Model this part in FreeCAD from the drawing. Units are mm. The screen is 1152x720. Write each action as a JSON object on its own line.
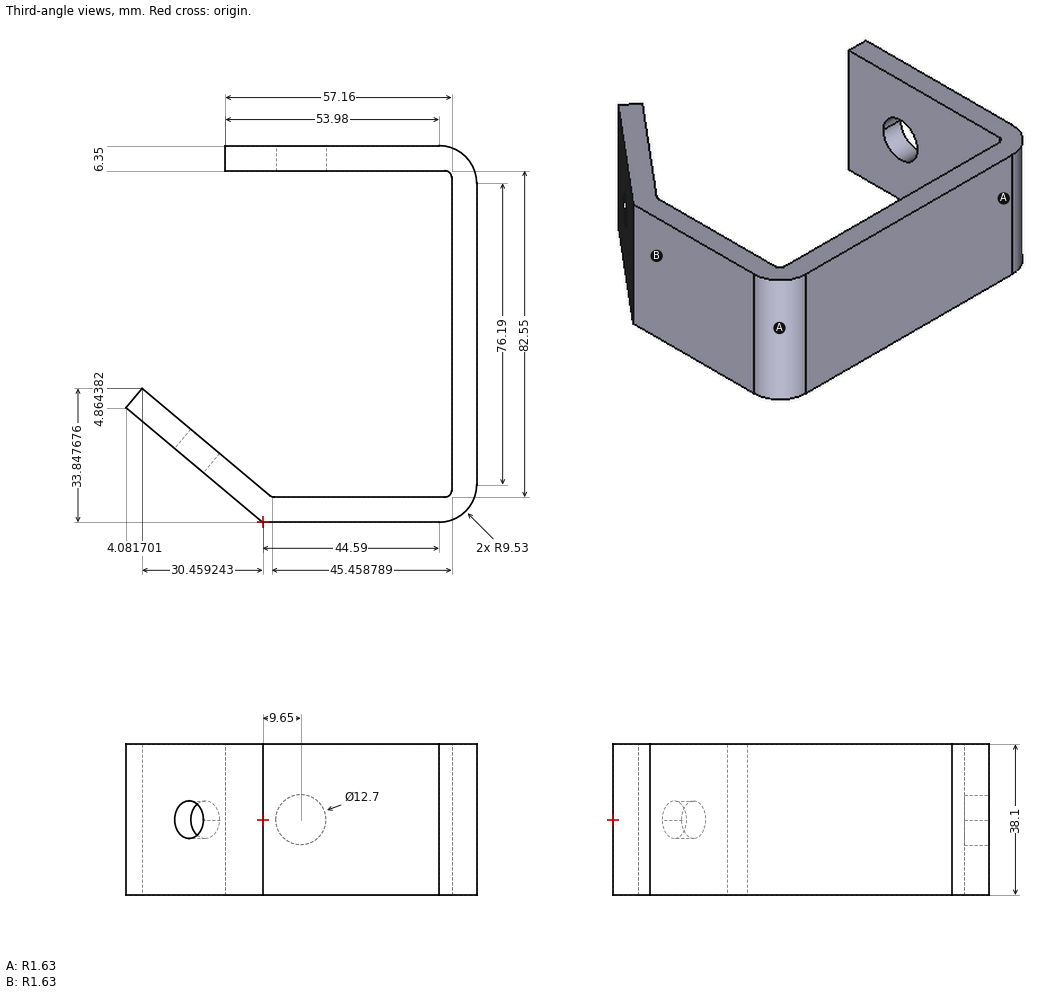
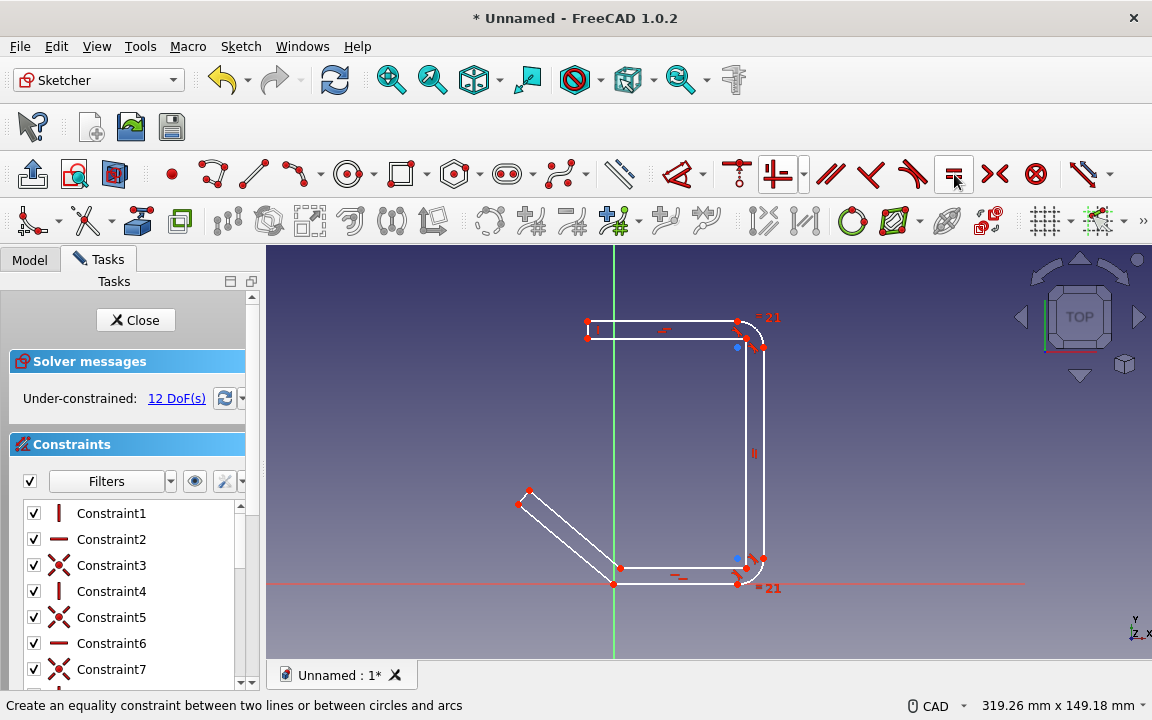
{"action": "key", "text": "d"}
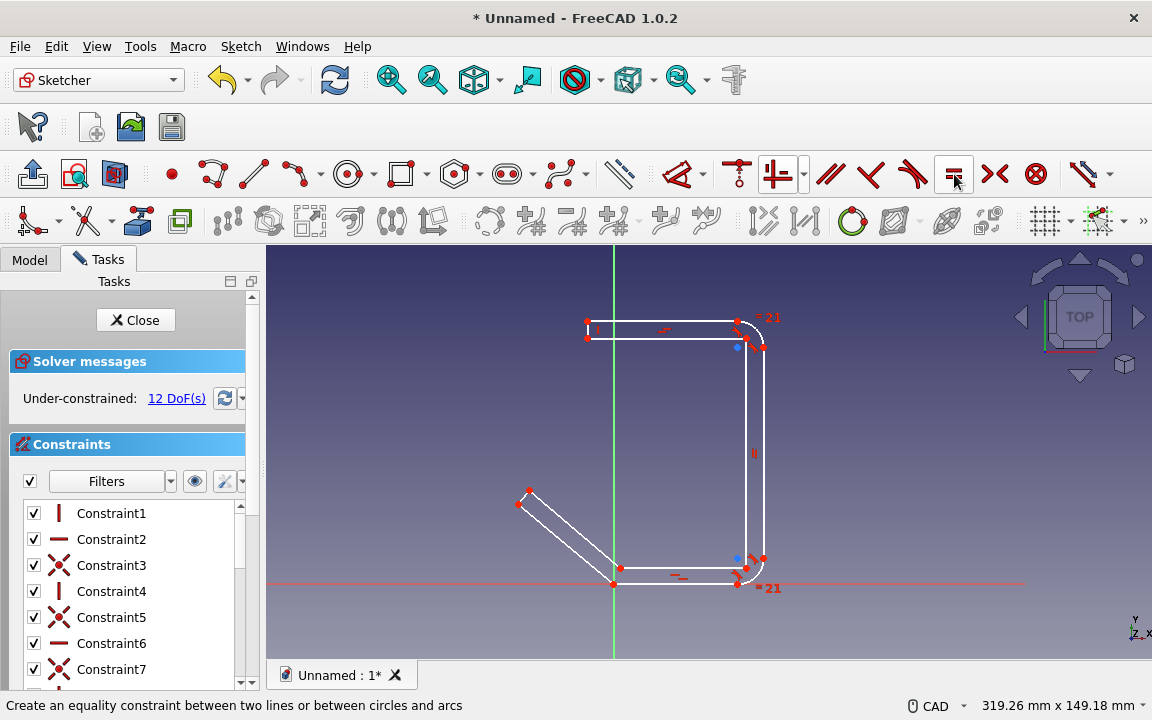
{"action": "scroll", "coordinate": [761, 335], "scroll_direction": "up", "scroll_amount": 3}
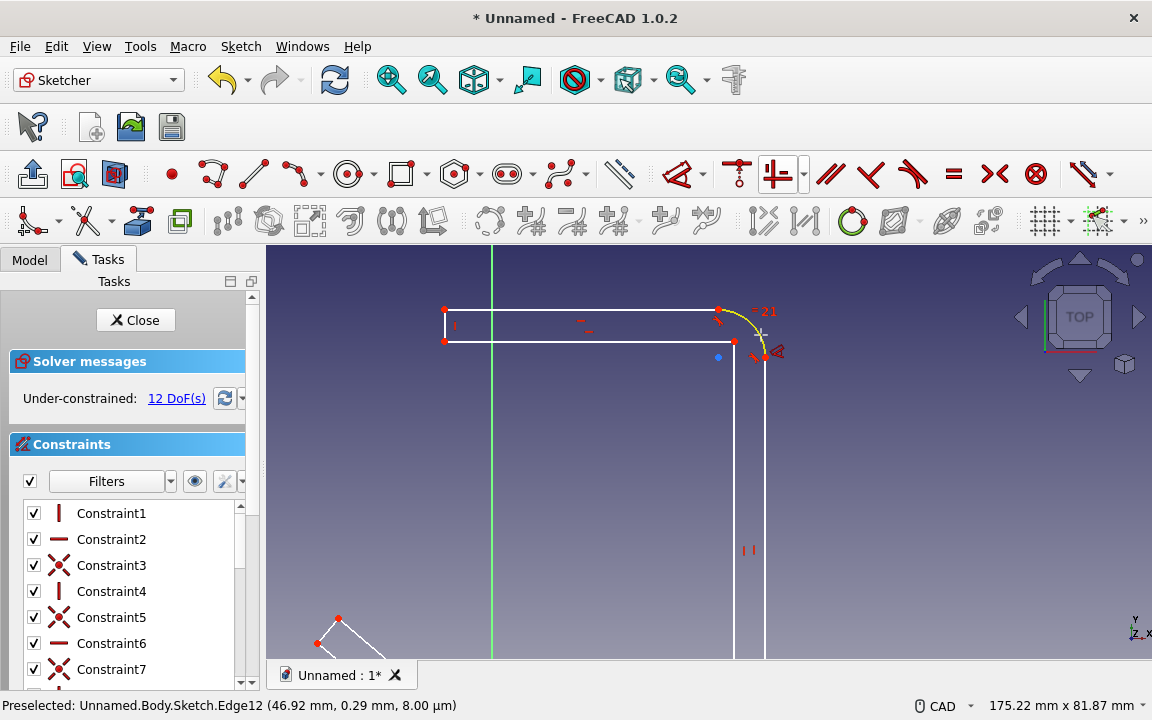
{"action": "left_click", "coordinate": [760, 336]}
{"action": "left_click", "coordinate": [789, 322]}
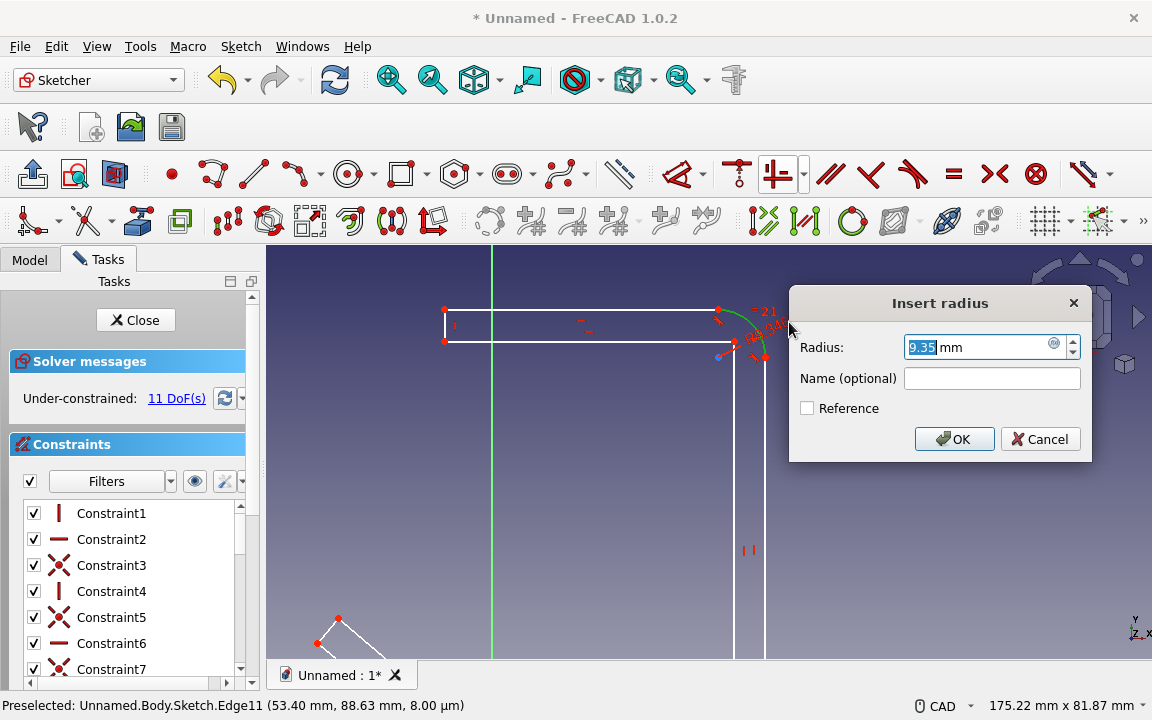
{"action": "type", "text": "9.53"}
{"action": "key", "text": "Return"}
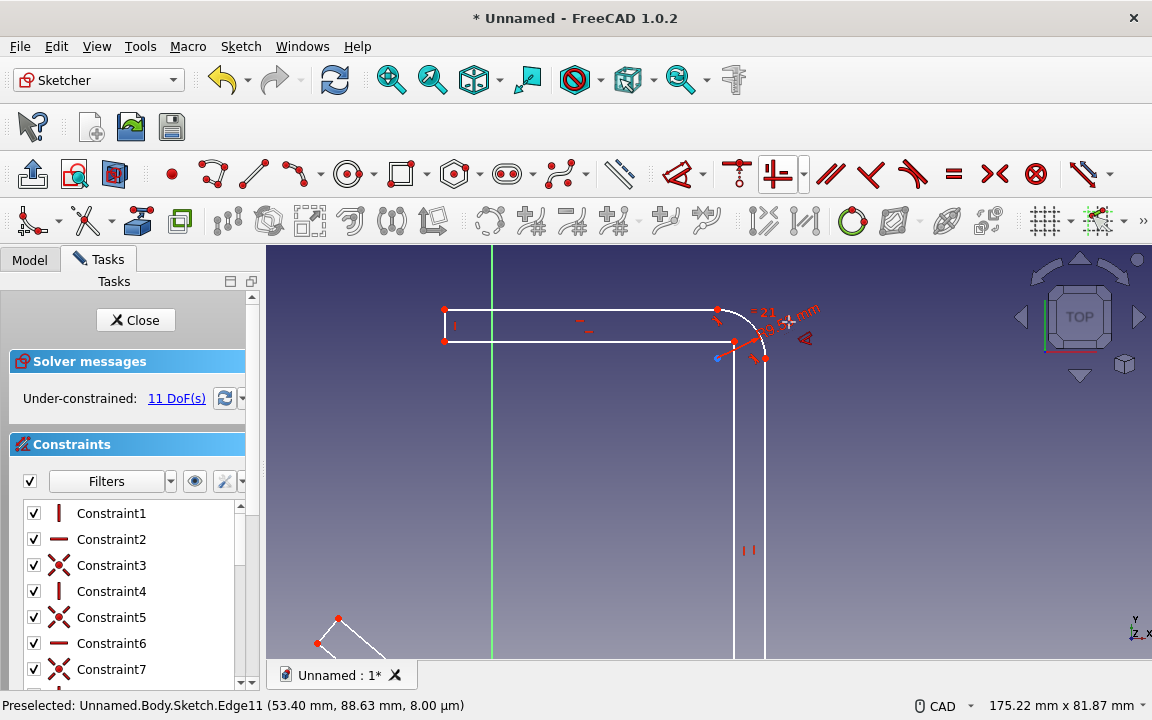
{"action": "scroll", "coordinate": [445, 319], "scroll_direction": "up", "scroll_amount": 2}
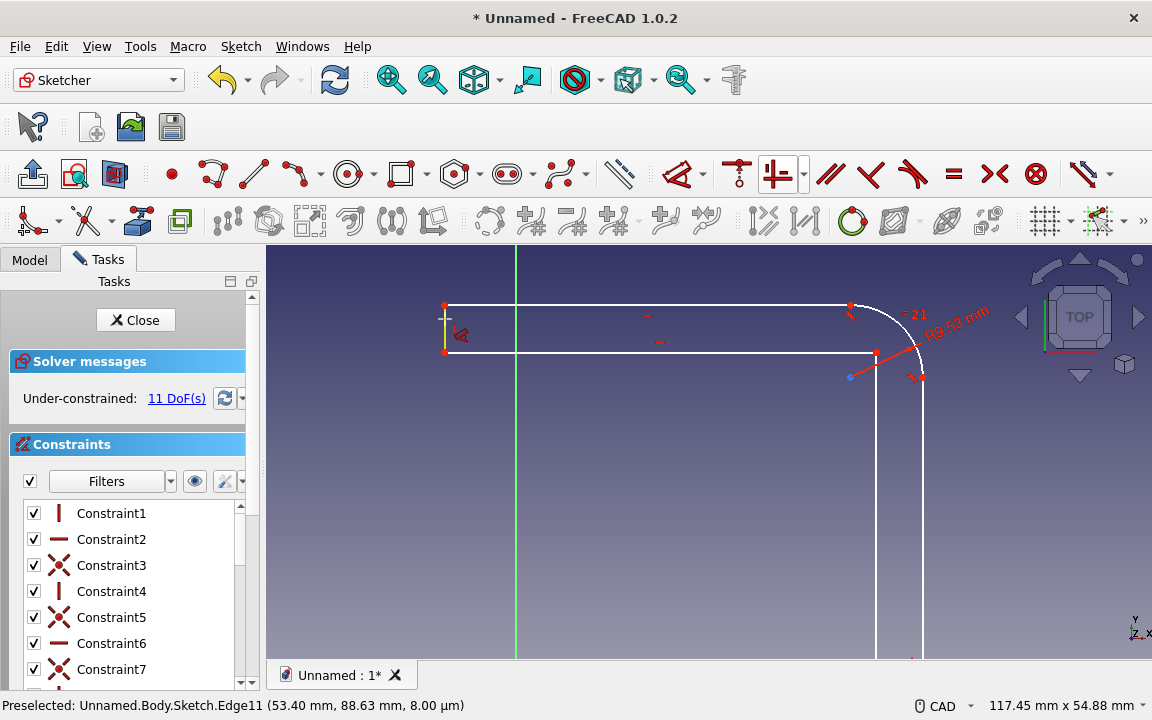
{"action": "left_click", "coordinate": [445, 319]}
{"action": "left_click", "coordinate": [411, 329]}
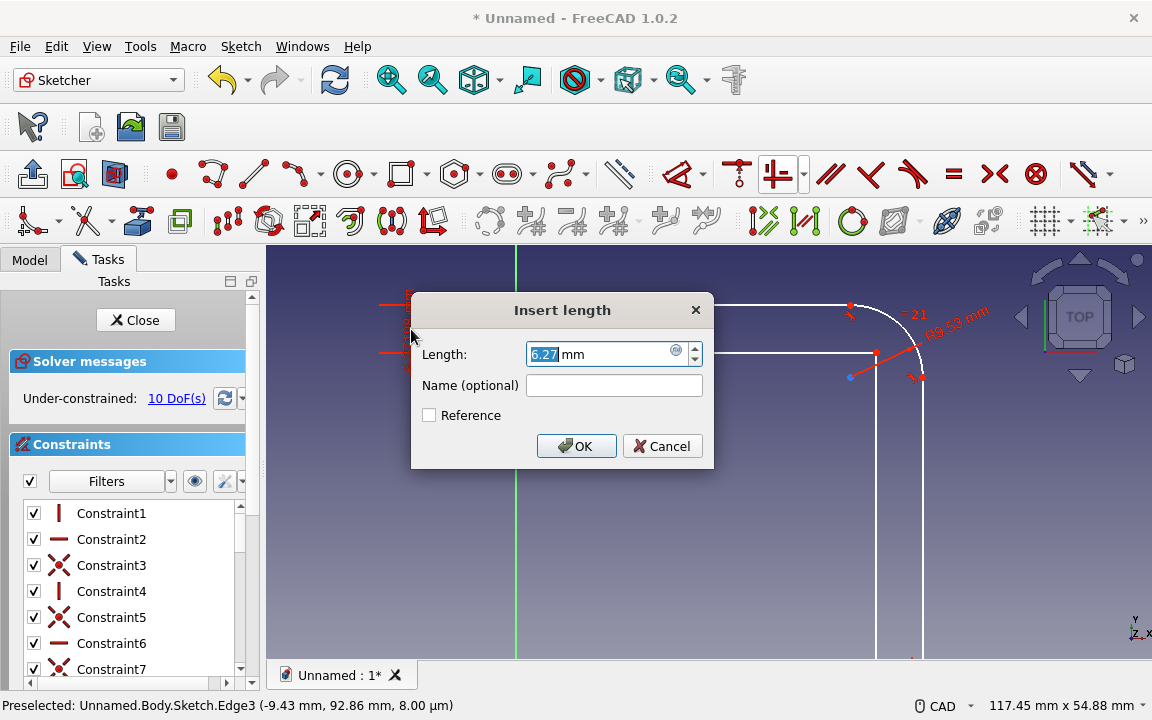
{"action": "type", "text": "6.35"}
{"action": "key", "text": "Return"}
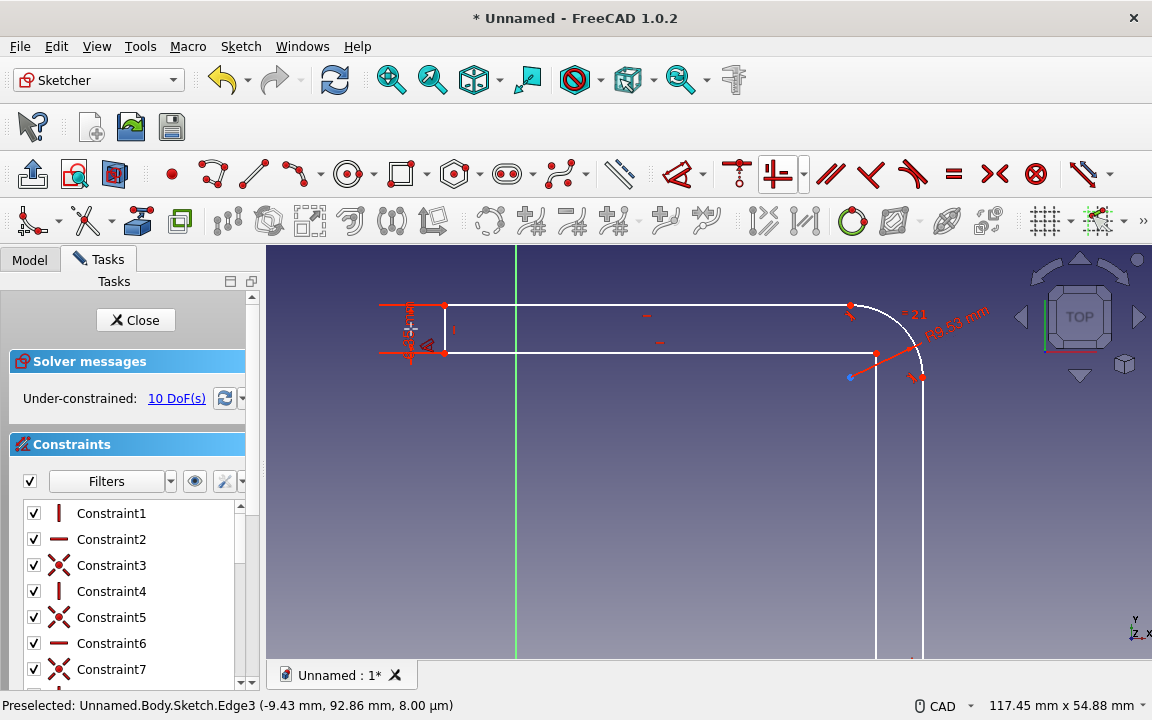
{"action": "left_click", "coordinate": [923, 549]}
{"action": "left_click", "coordinate": [957, 504]}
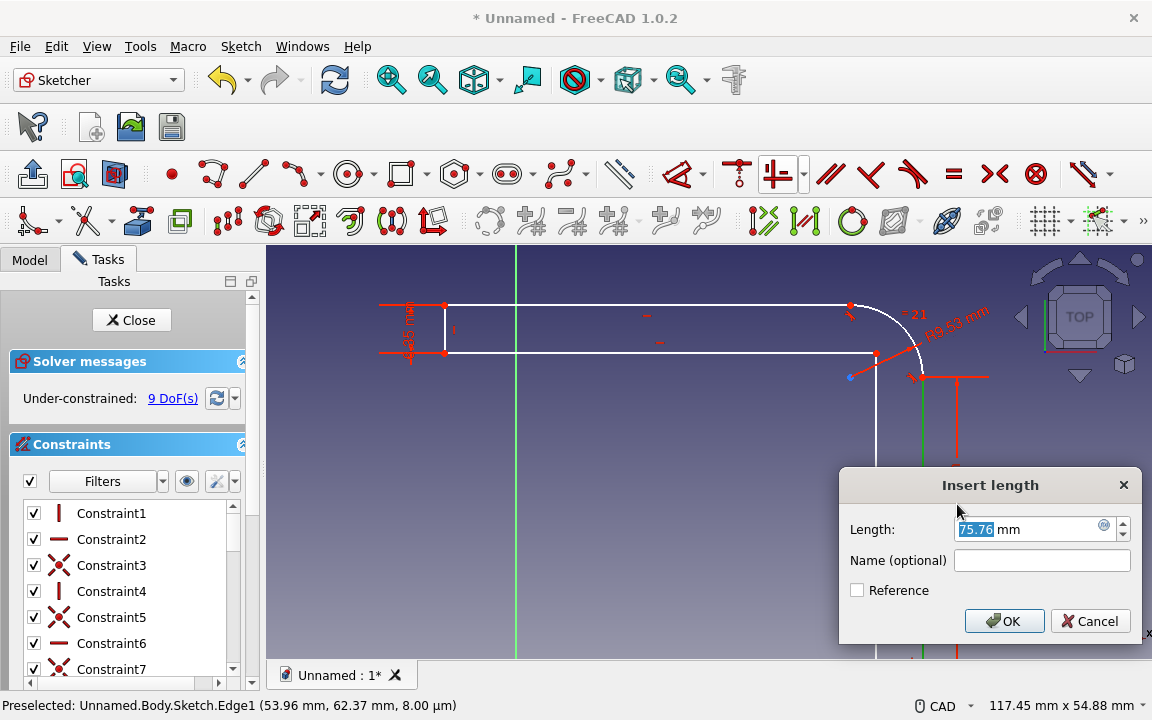
{"action": "type", "text": "76.19"}
{"action": "key", "text": "Return"}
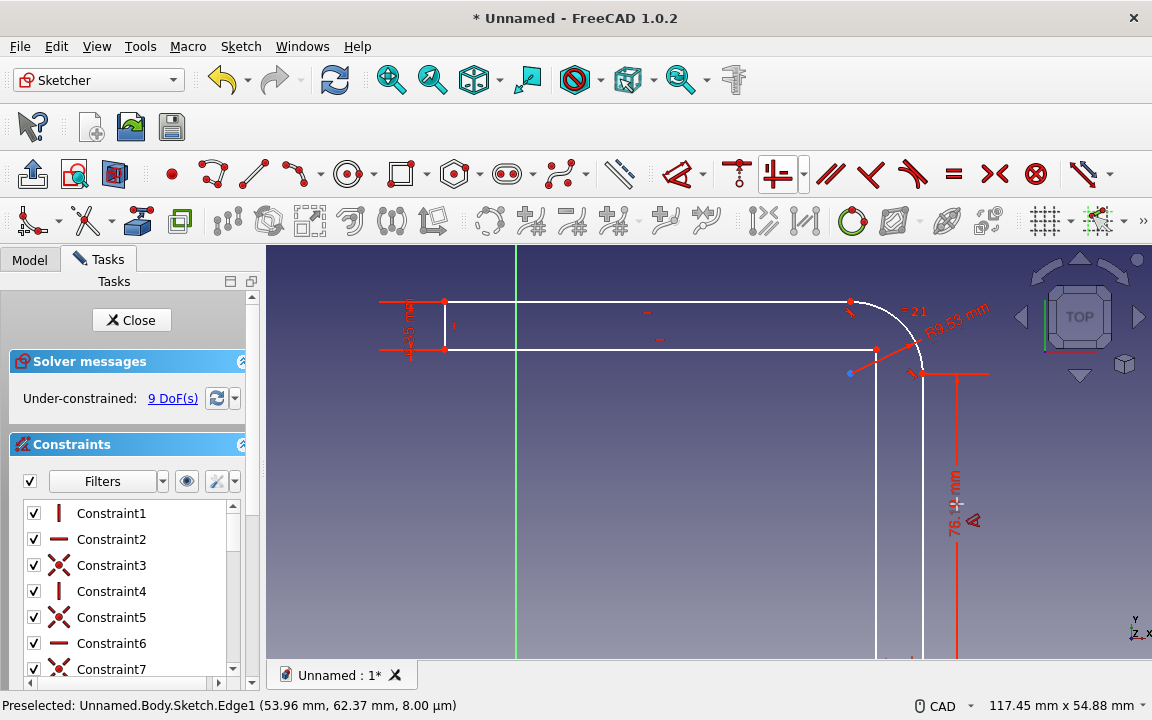
{"action": "left_click", "coordinate": [729, 302]}
{"action": "left_click", "coordinate": [648, 336]}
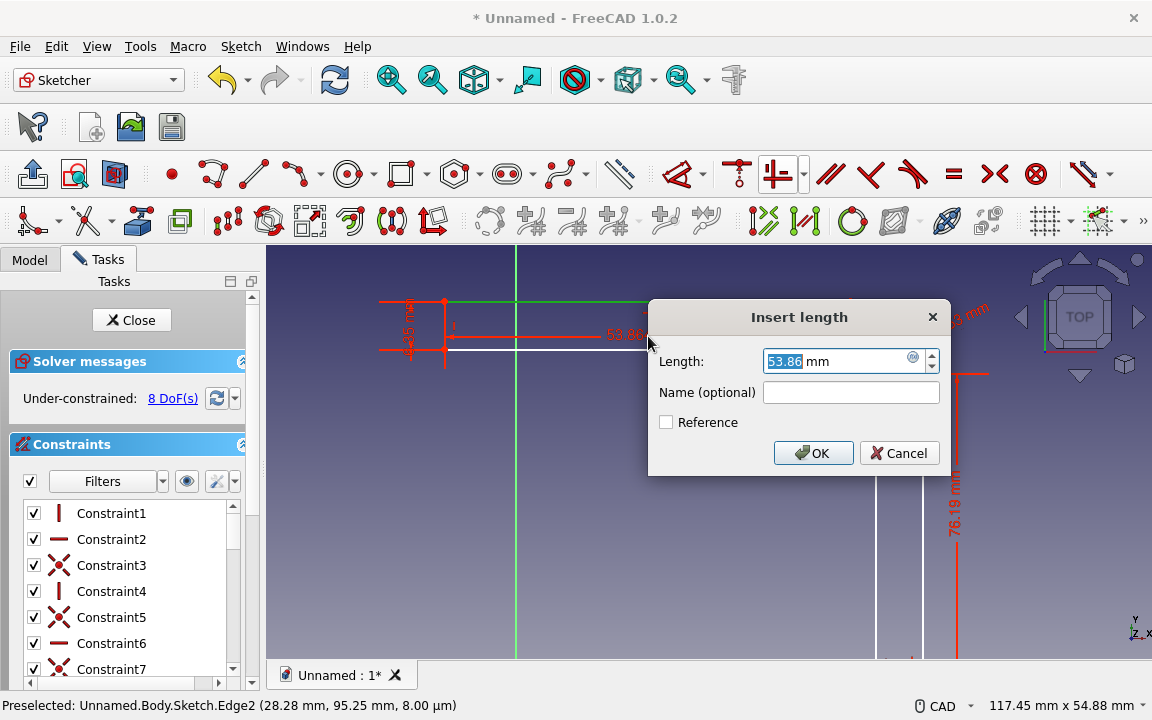
{"action": "type", "text": "53.98"}
{"action": "key", "text": "Return"}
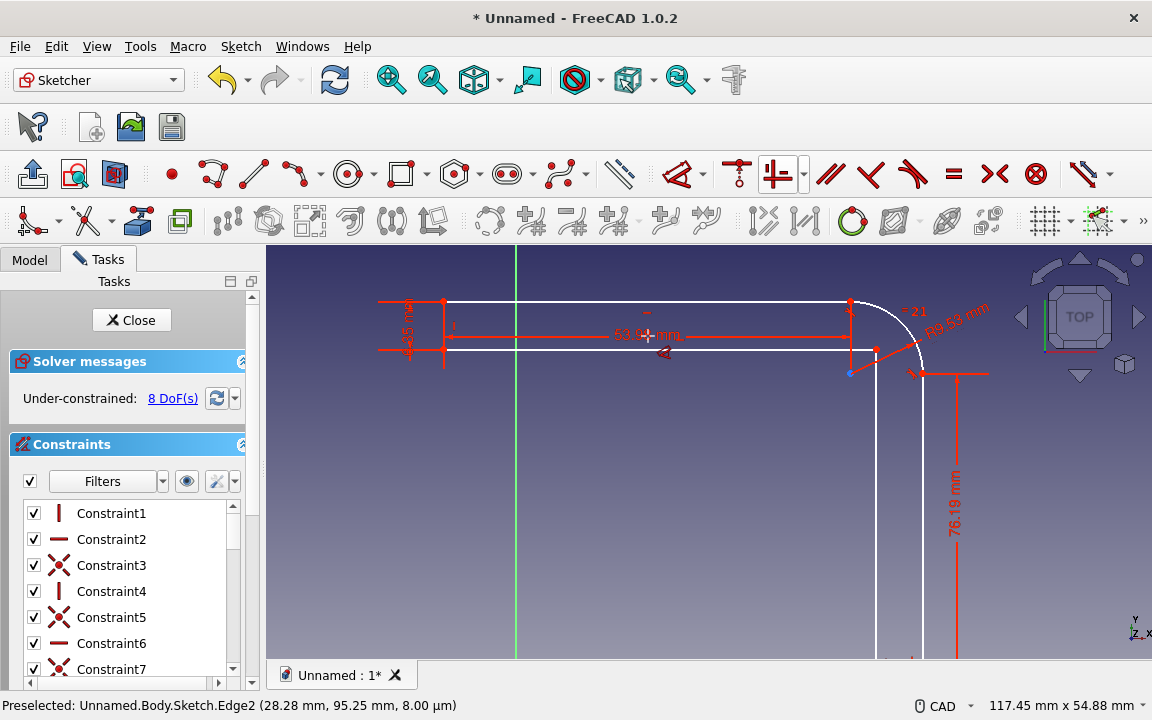
{"action": "left_click", "coordinate": [573, 350]}
{"action": "left_click", "coordinate": [660, 316]}